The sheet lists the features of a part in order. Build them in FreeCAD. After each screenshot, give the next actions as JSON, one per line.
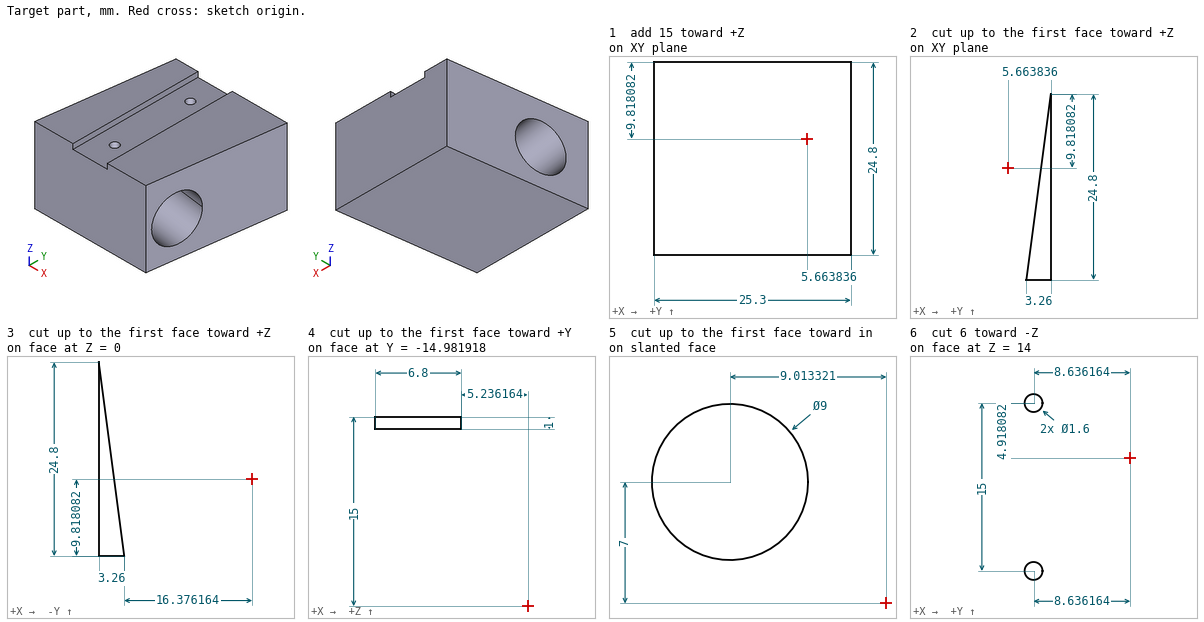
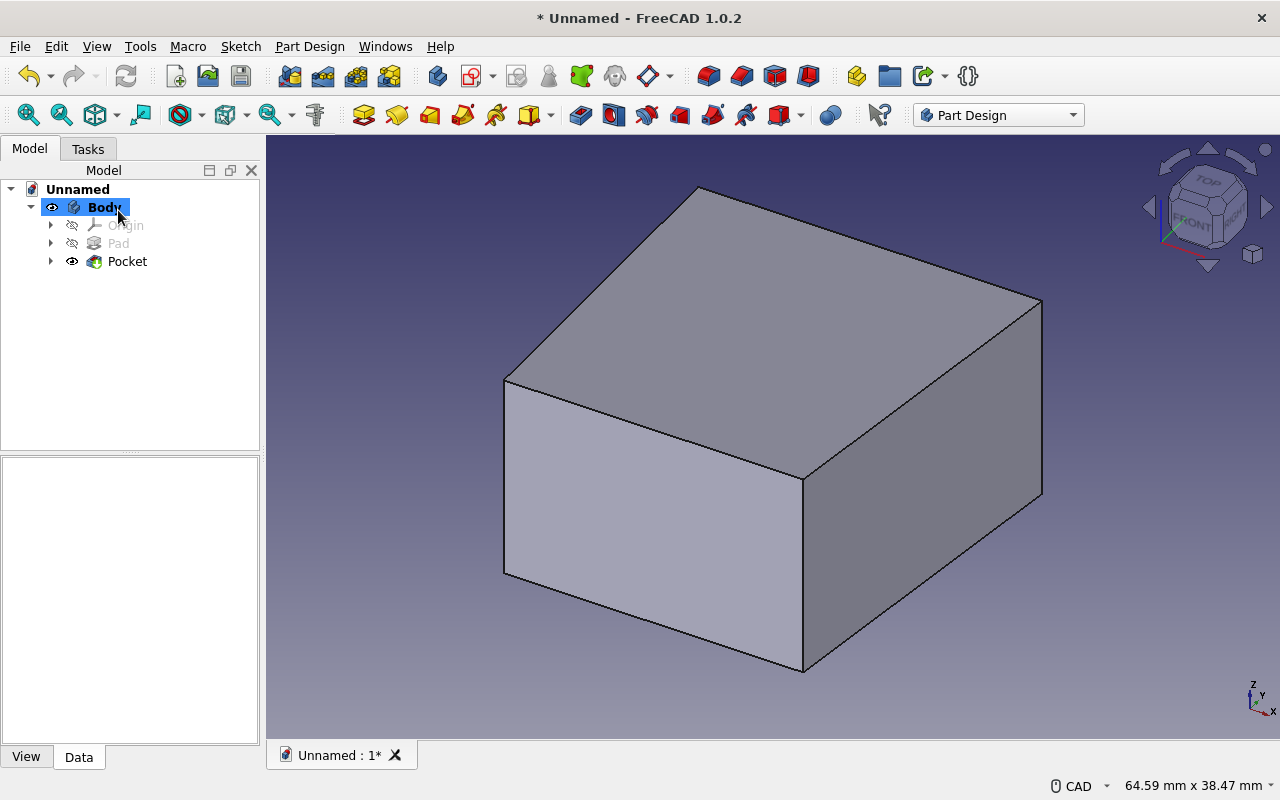
{"action": "key", "text": "5"}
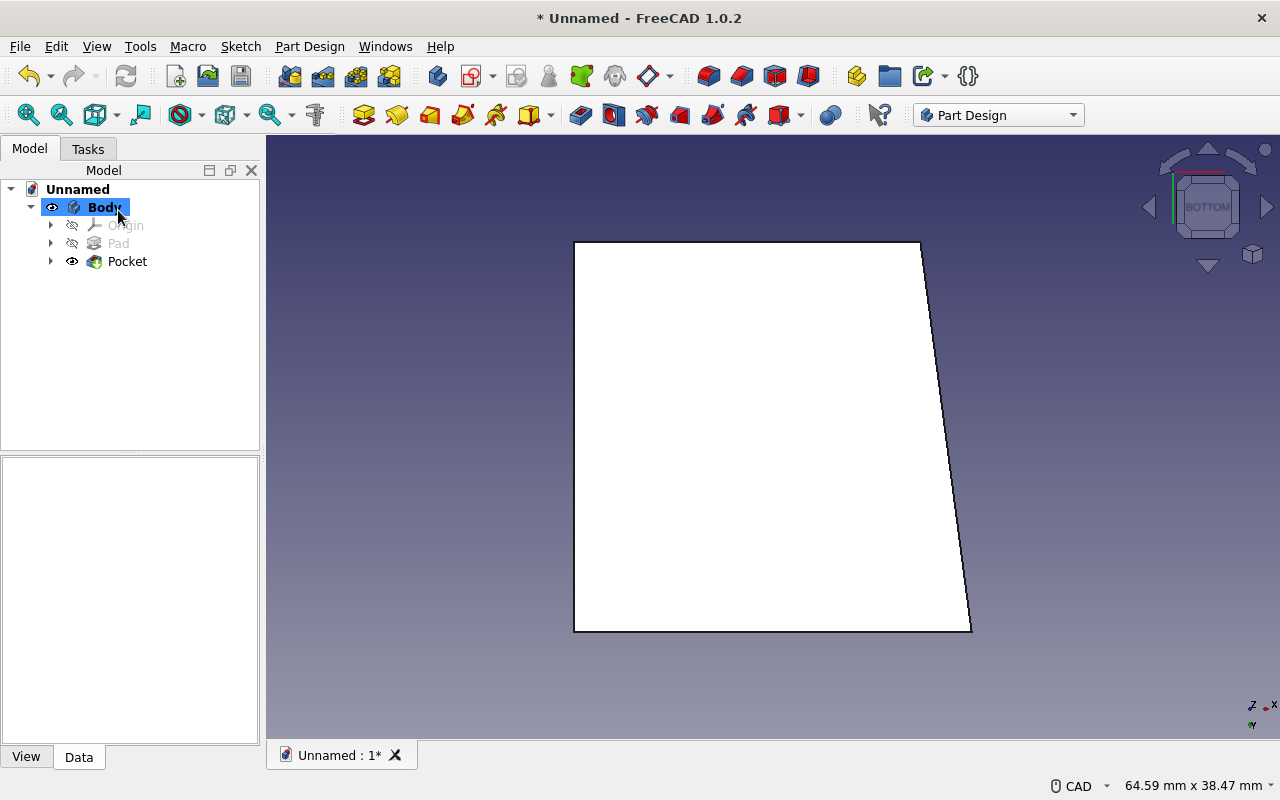
{"action": "left_click", "coordinate": [773, 436]}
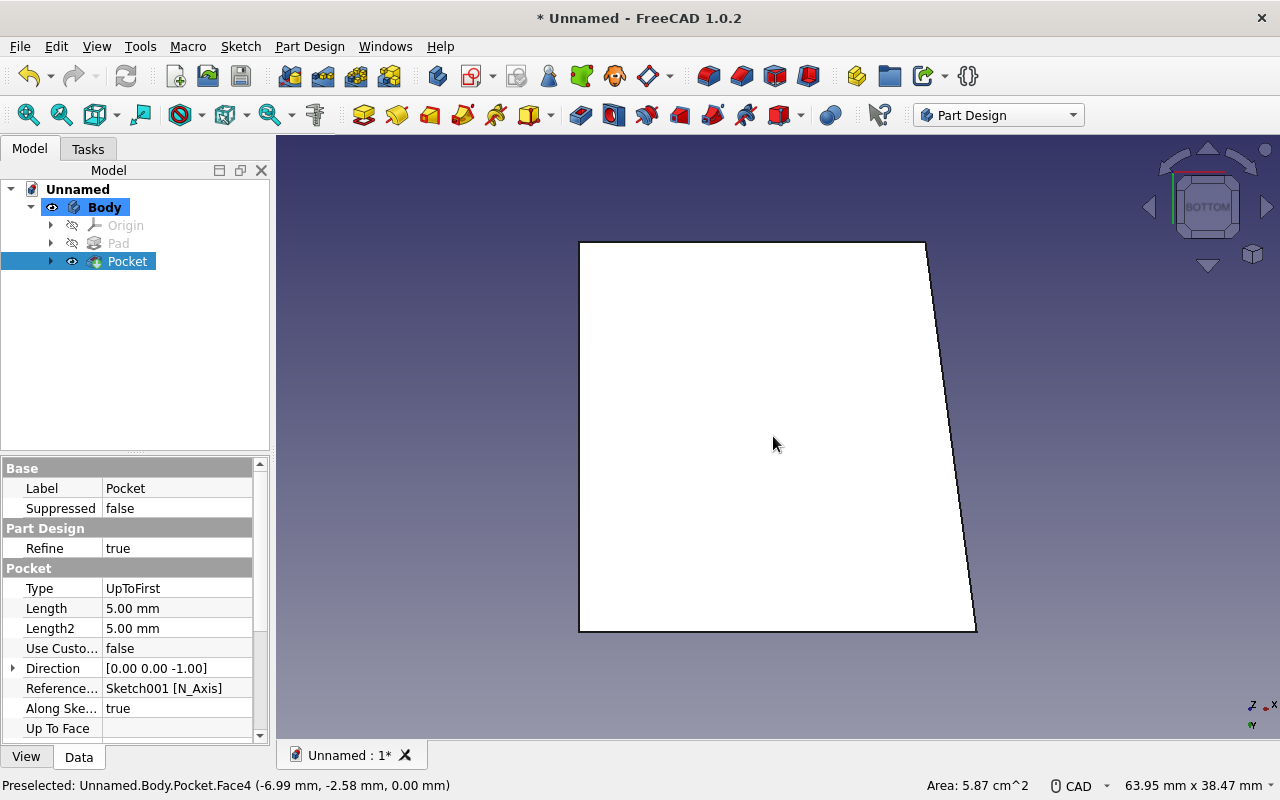
{"action": "left_click", "coordinate": [470, 76]}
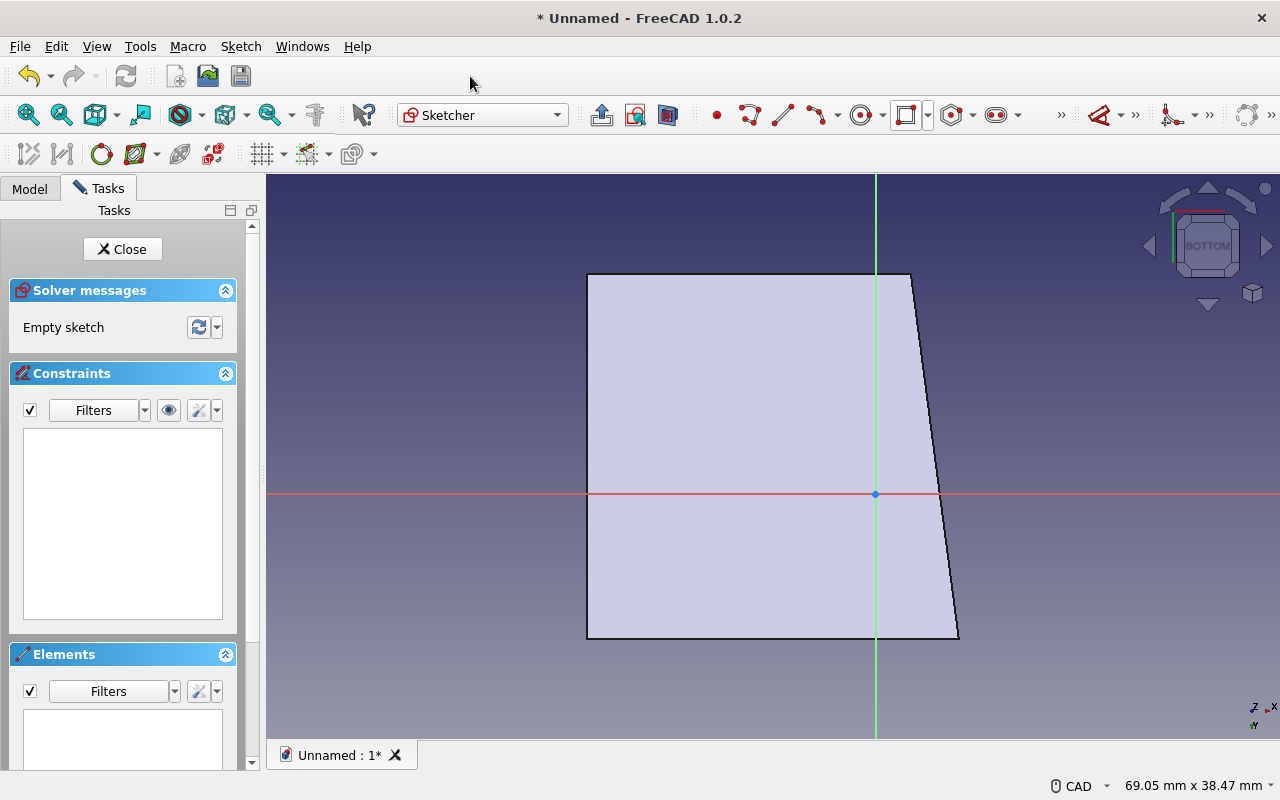
{"action": "left_click", "coordinate": [750, 116]}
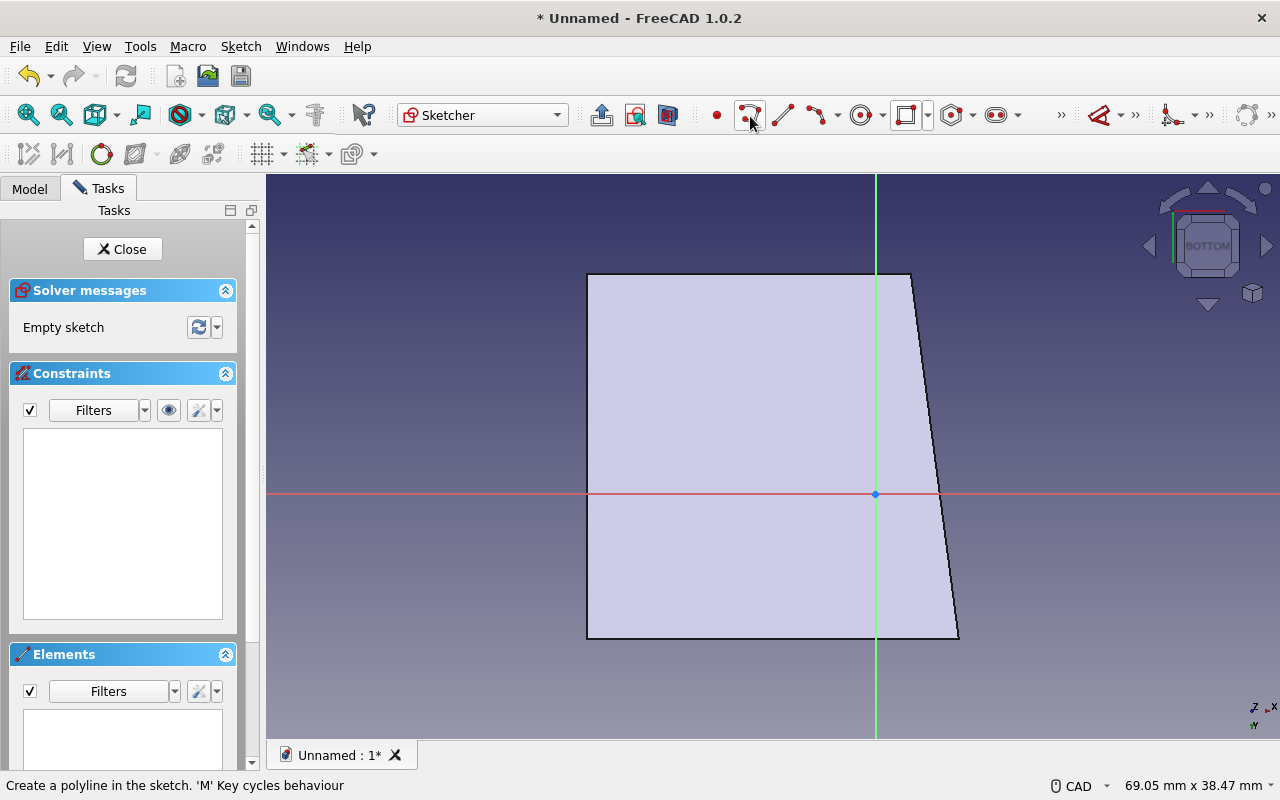
{"action": "left_click", "coordinate": [635, 639]}
{"action": "left_click", "coordinate": [587, 274]}
{"action": "left_click", "coordinate": [587, 639]}
{"action": "left_click", "coordinate": [635, 640]}
{"action": "key", "text": "Escape"}
{"action": "key", "text": "Escape"}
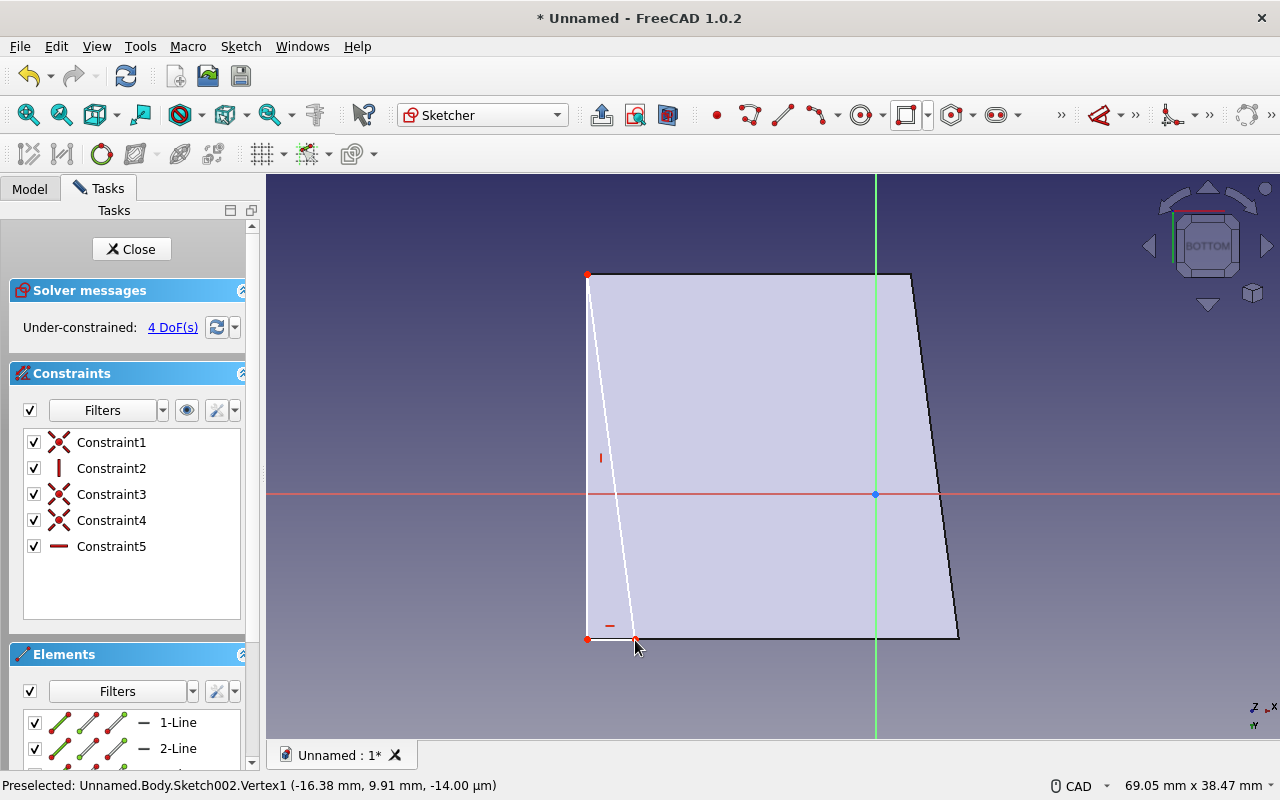
{"action": "left_click", "coordinate": [1098, 116]}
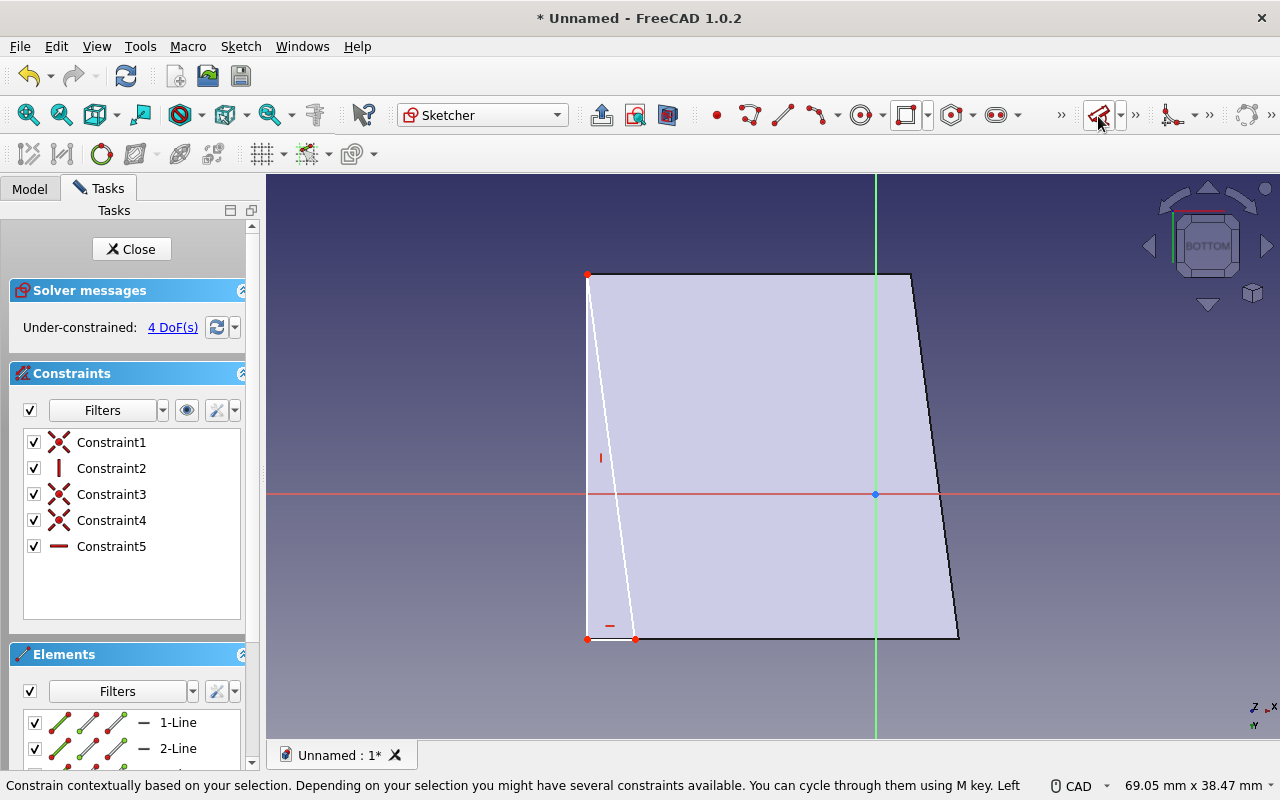
{"action": "left_click", "coordinate": [587, 385]}
{"action": "left_click", "coordinate": [553, 457]}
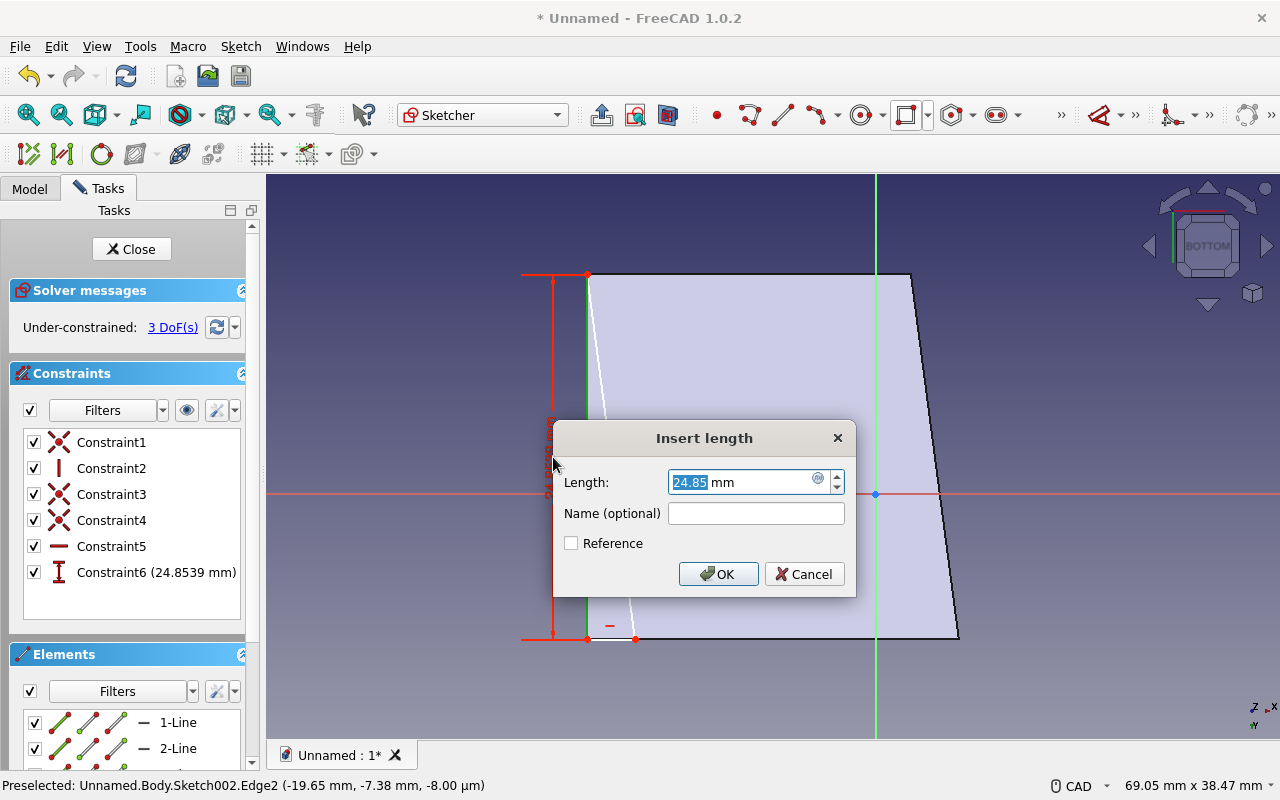
{"action": "type", "text": "24.8"}
{"action": "key", "text": "Return"}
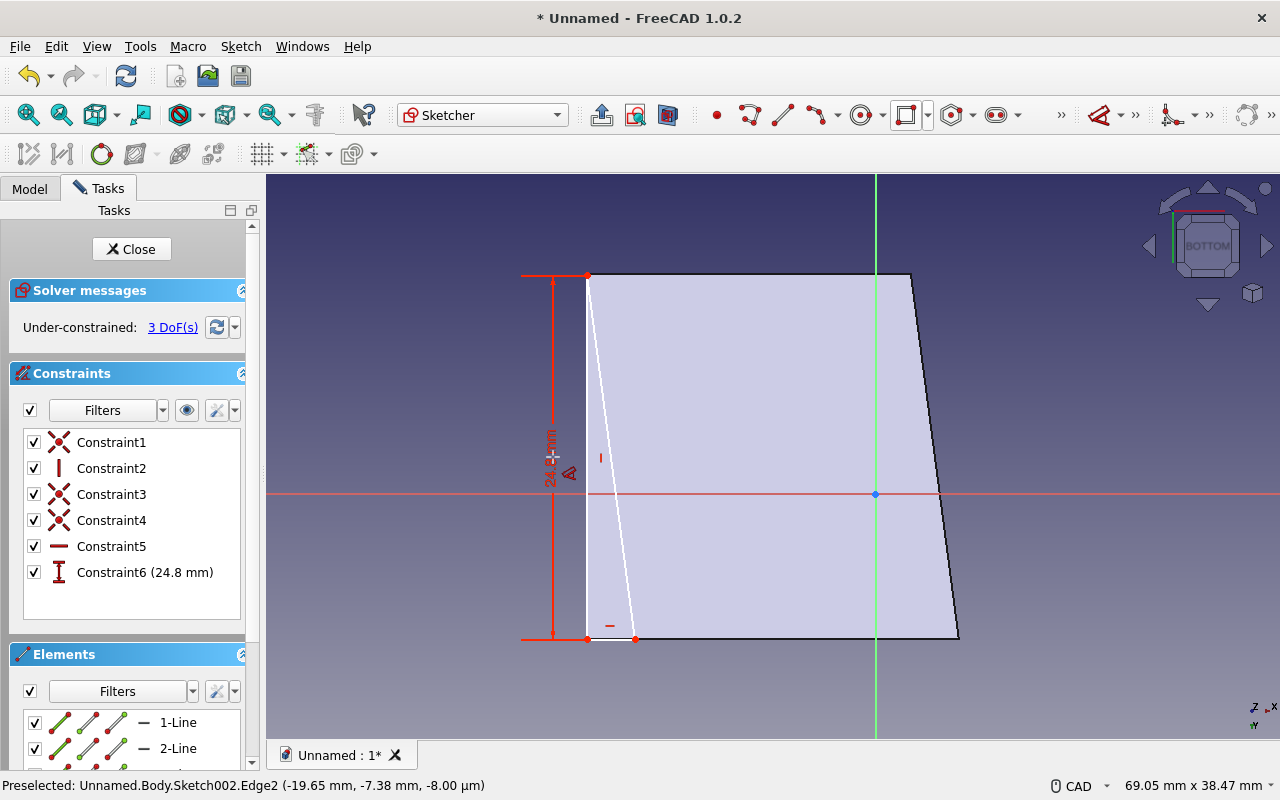
{"action": "left_click", "coordinate": [601, 640]}
{"action": "left_click", "coordinate": [611, 674]}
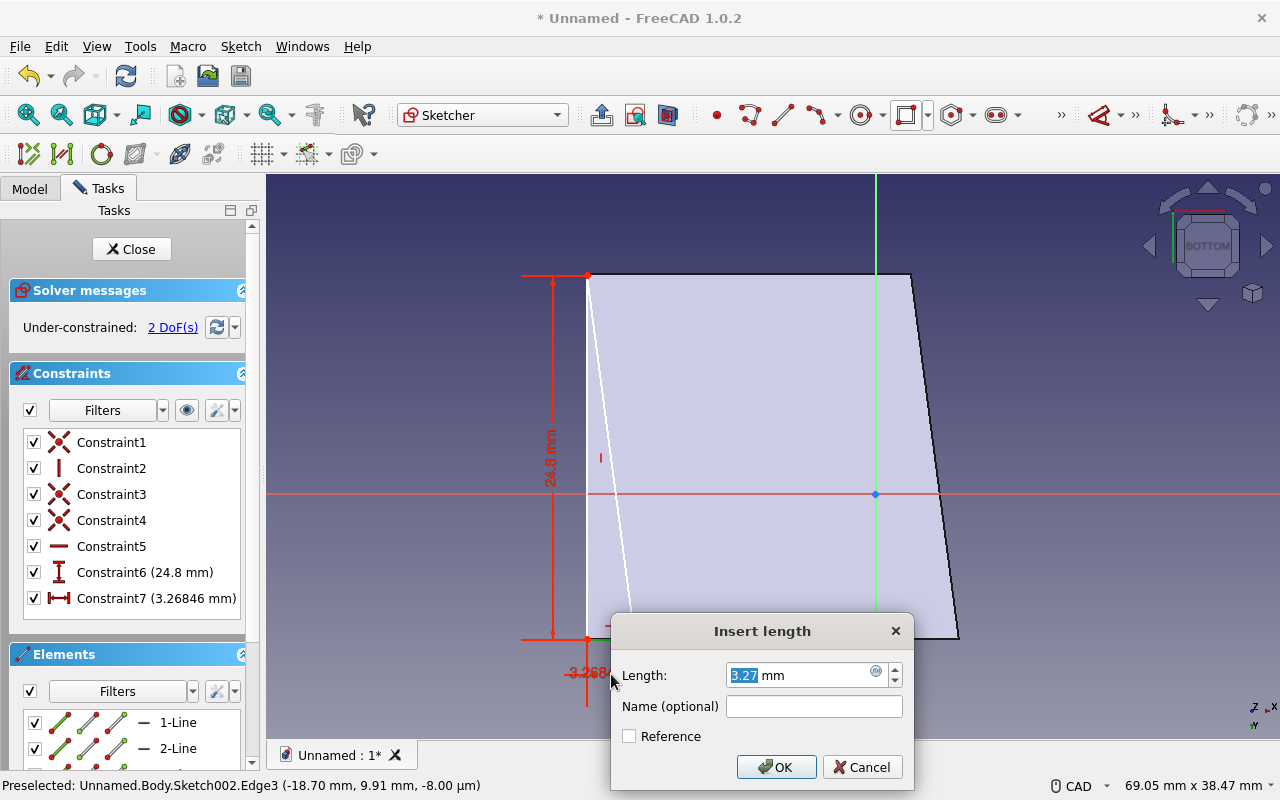
{"action": "type", "text": "3.26"}
{"action": "key", "text": "Return"}